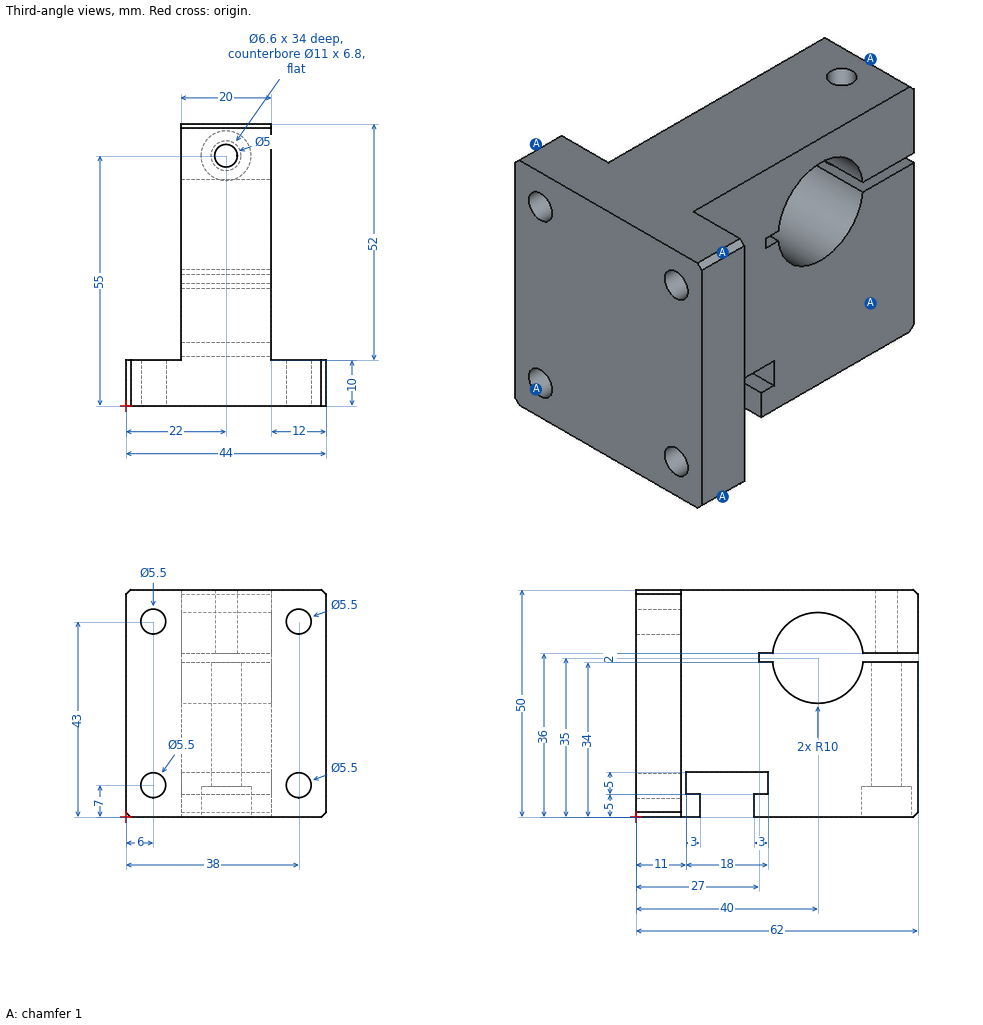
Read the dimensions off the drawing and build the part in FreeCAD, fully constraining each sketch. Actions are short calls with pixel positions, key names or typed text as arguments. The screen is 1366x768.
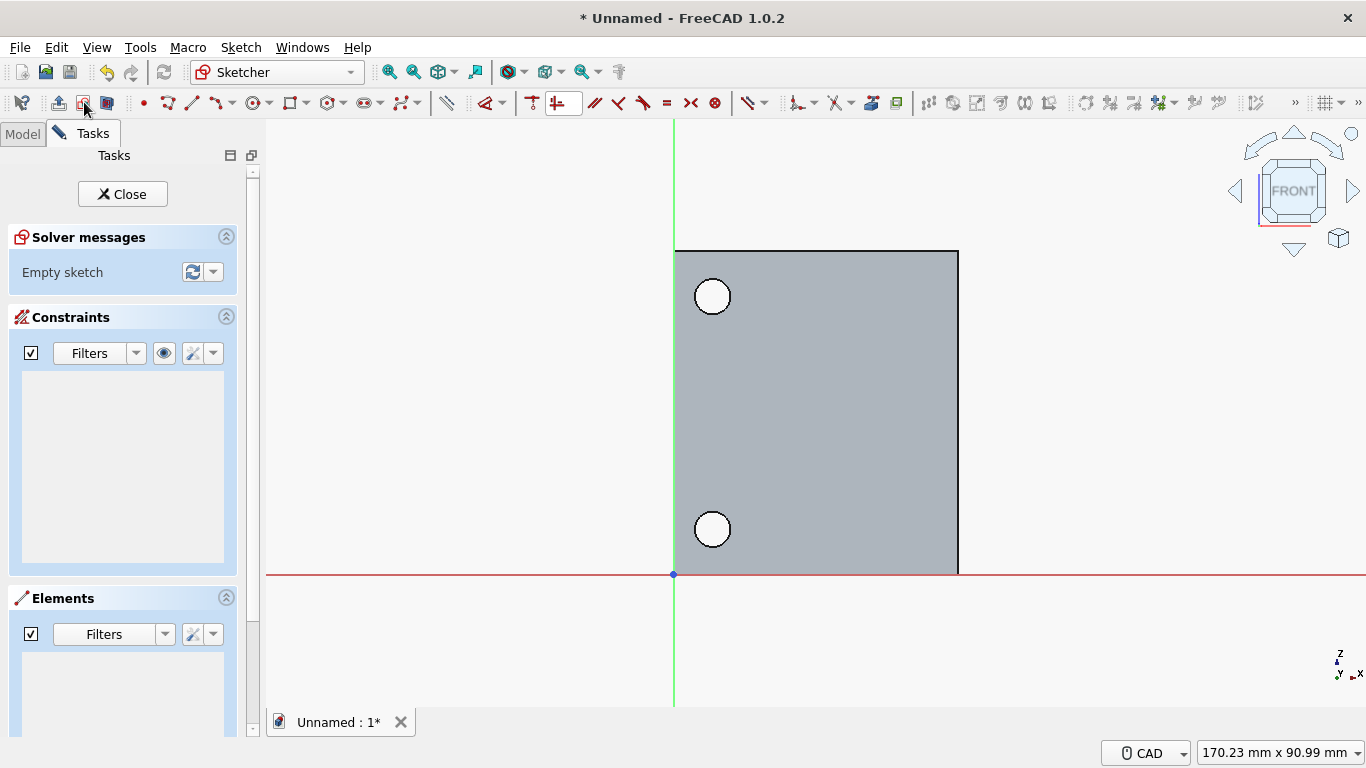
scroll(937, 285, up, 12)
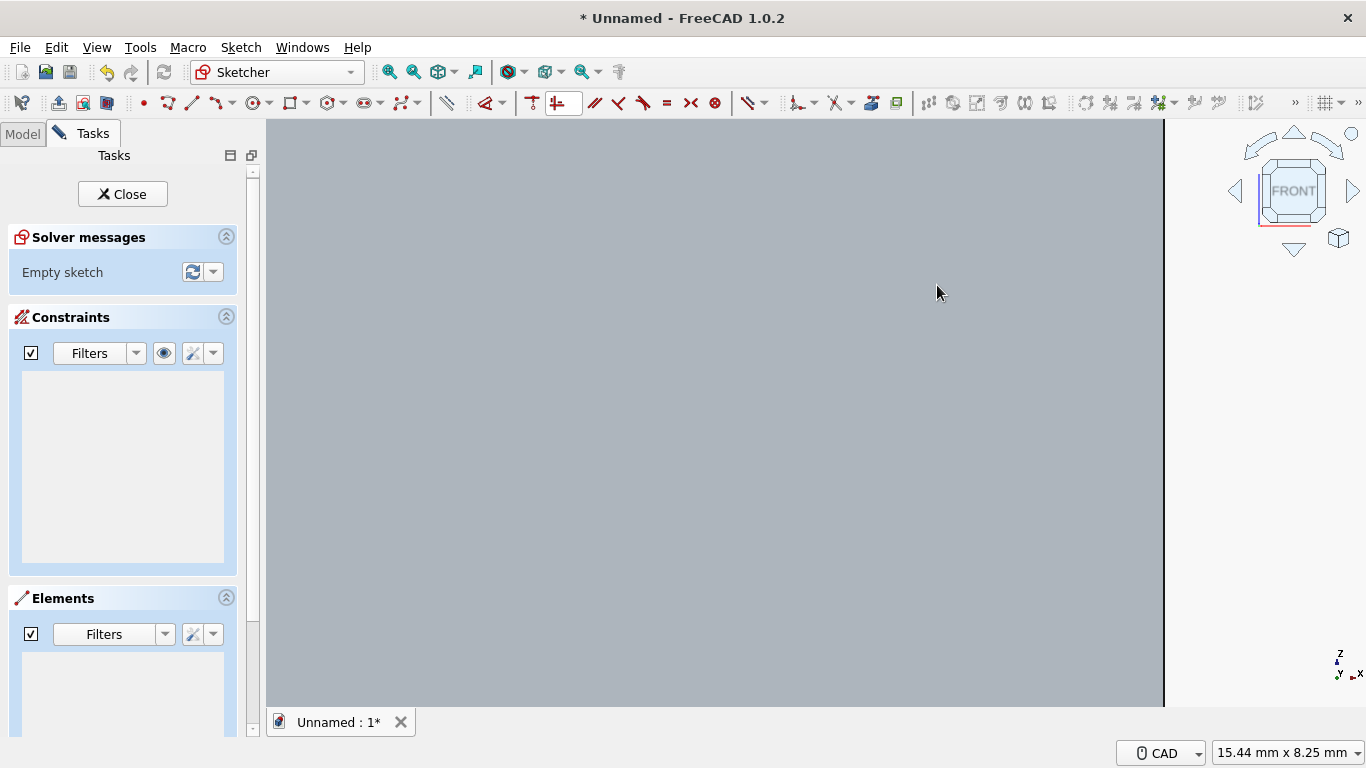
click(254, 104)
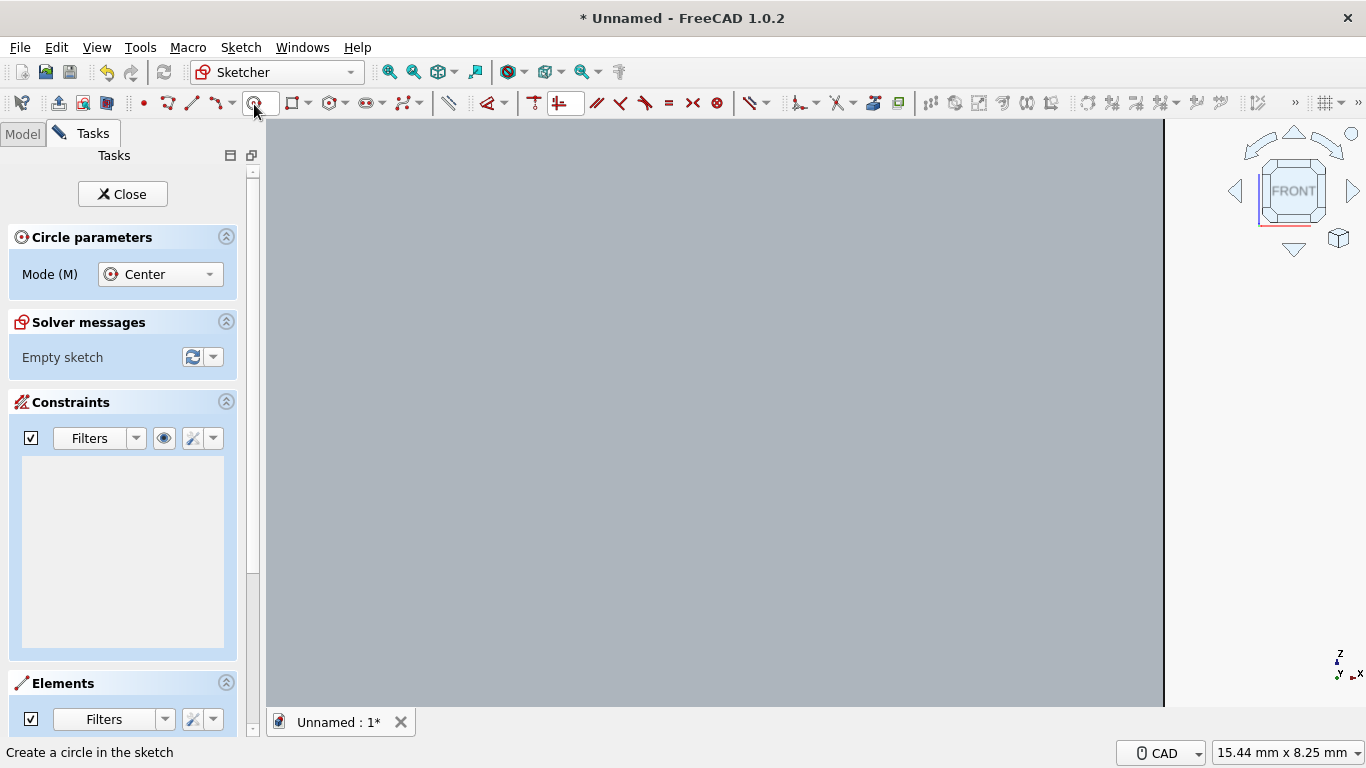
click(737, 411)
move(875, 272)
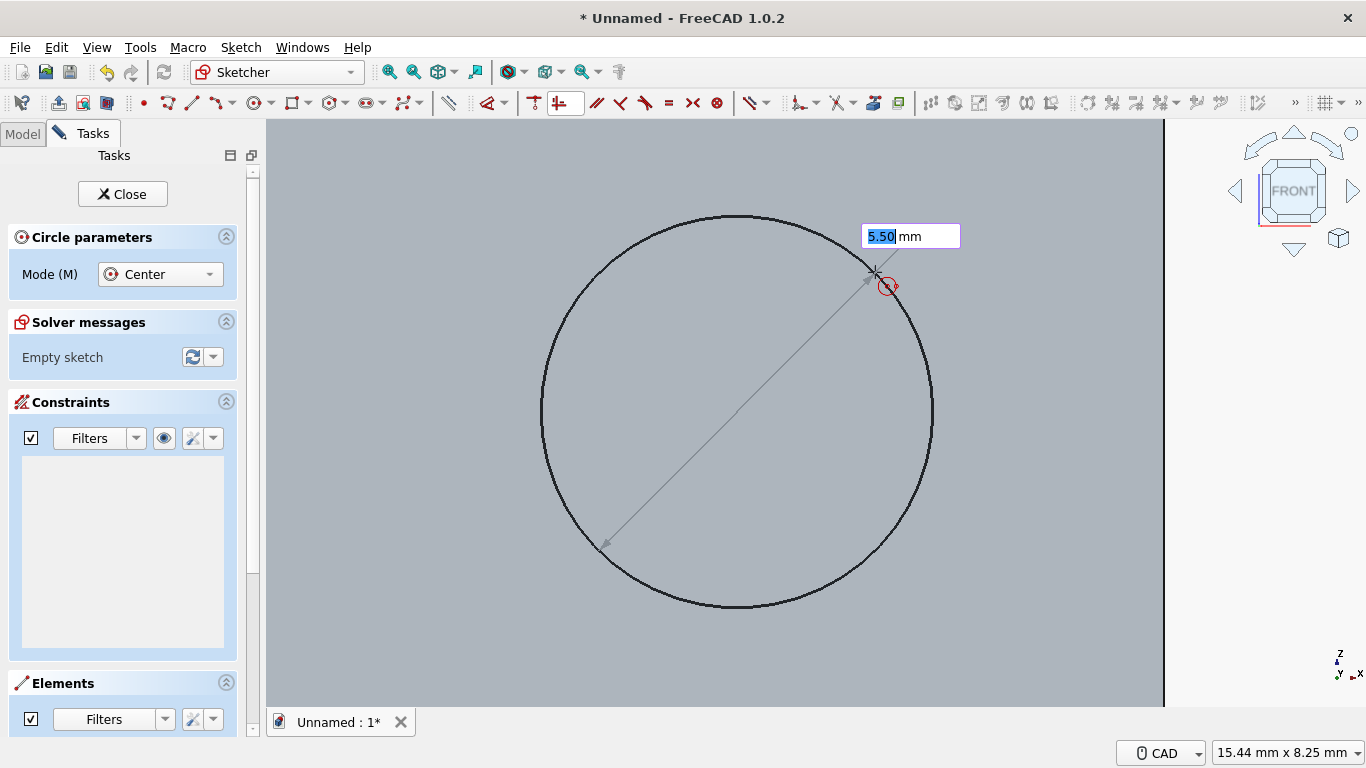
text(5.5)
key(Return)
key(Escape)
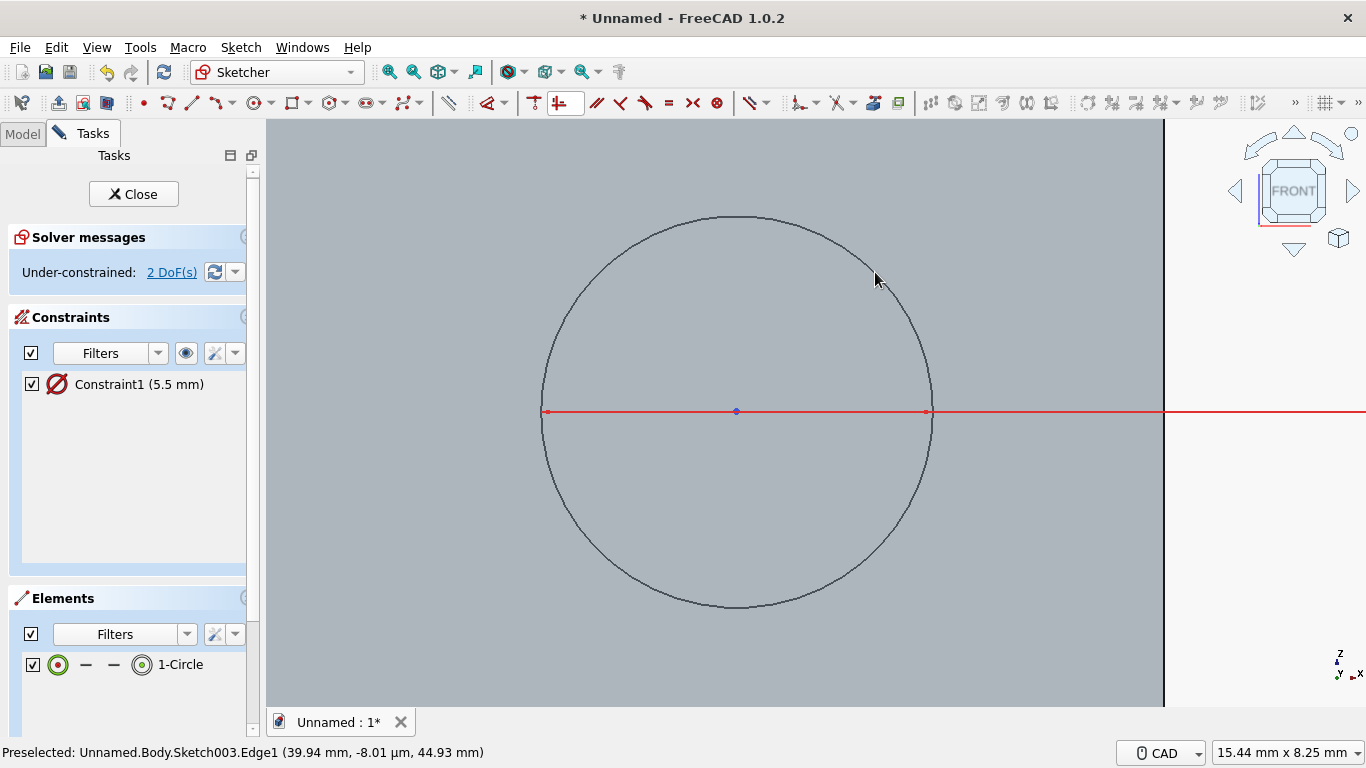
click(488, 104)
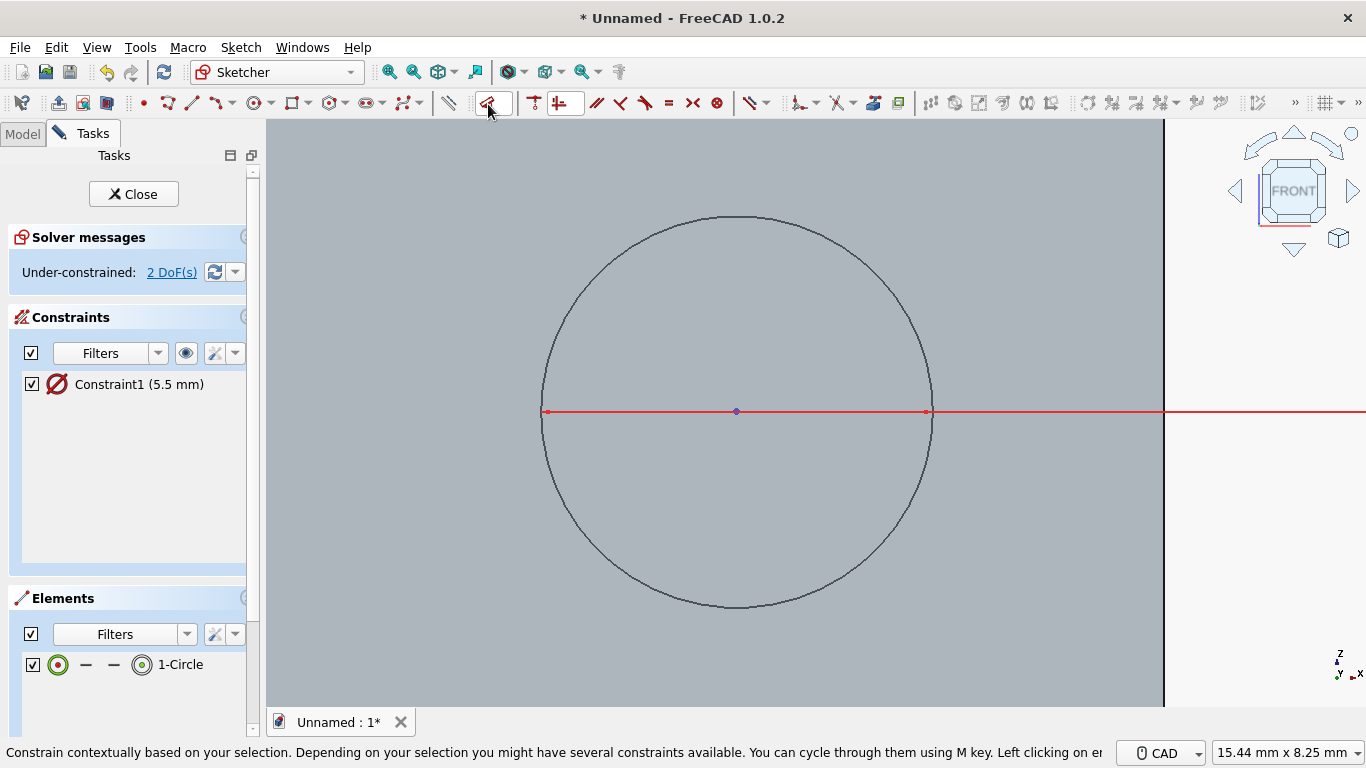
click(737, 412)
click(515, 378)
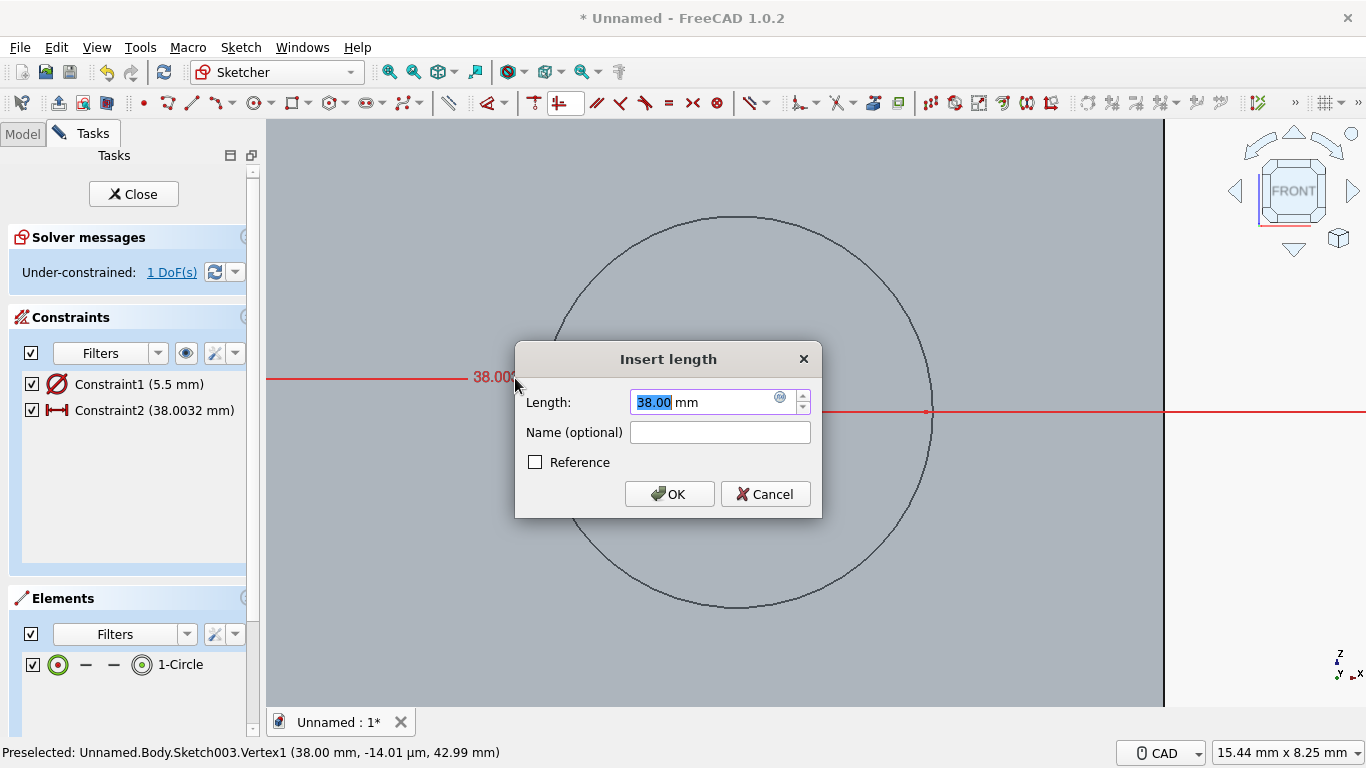
text(38)
key(Return)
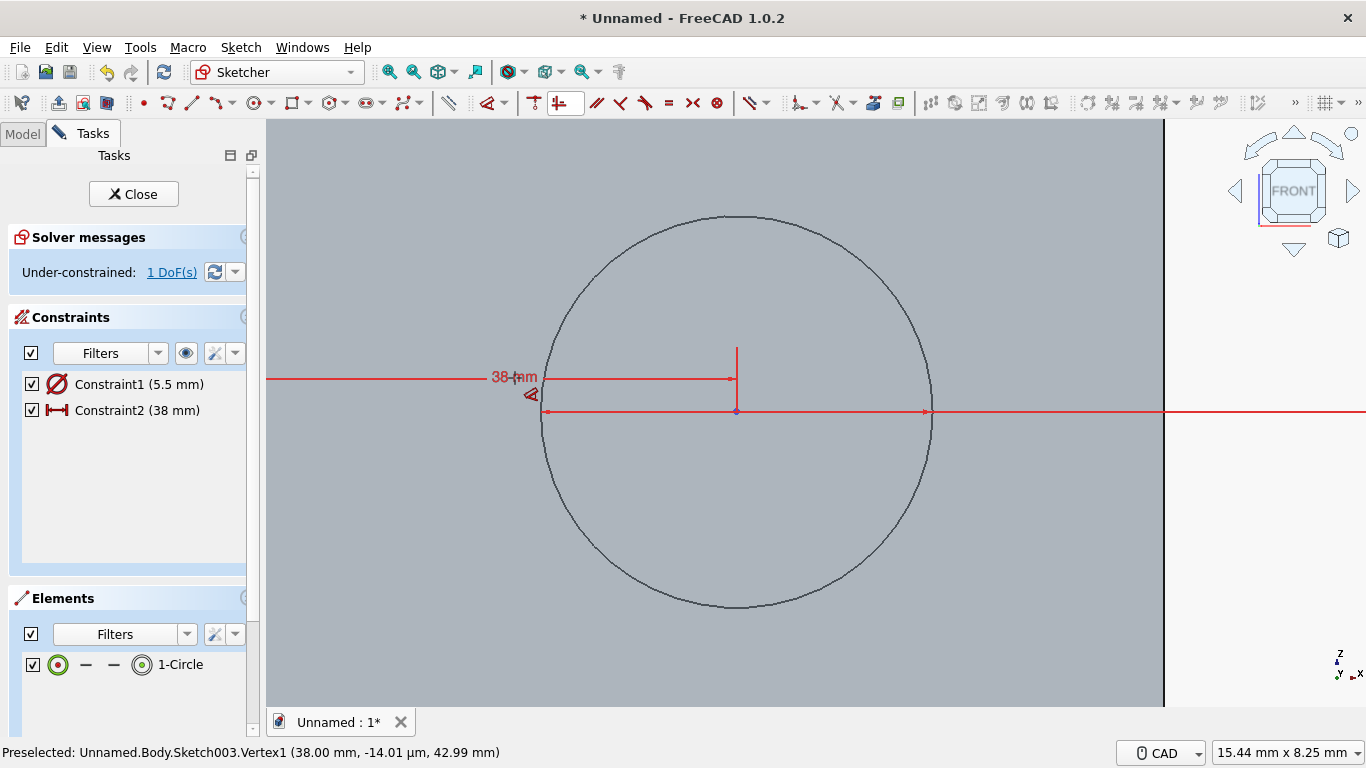
click(737, 412)
click(771, 546)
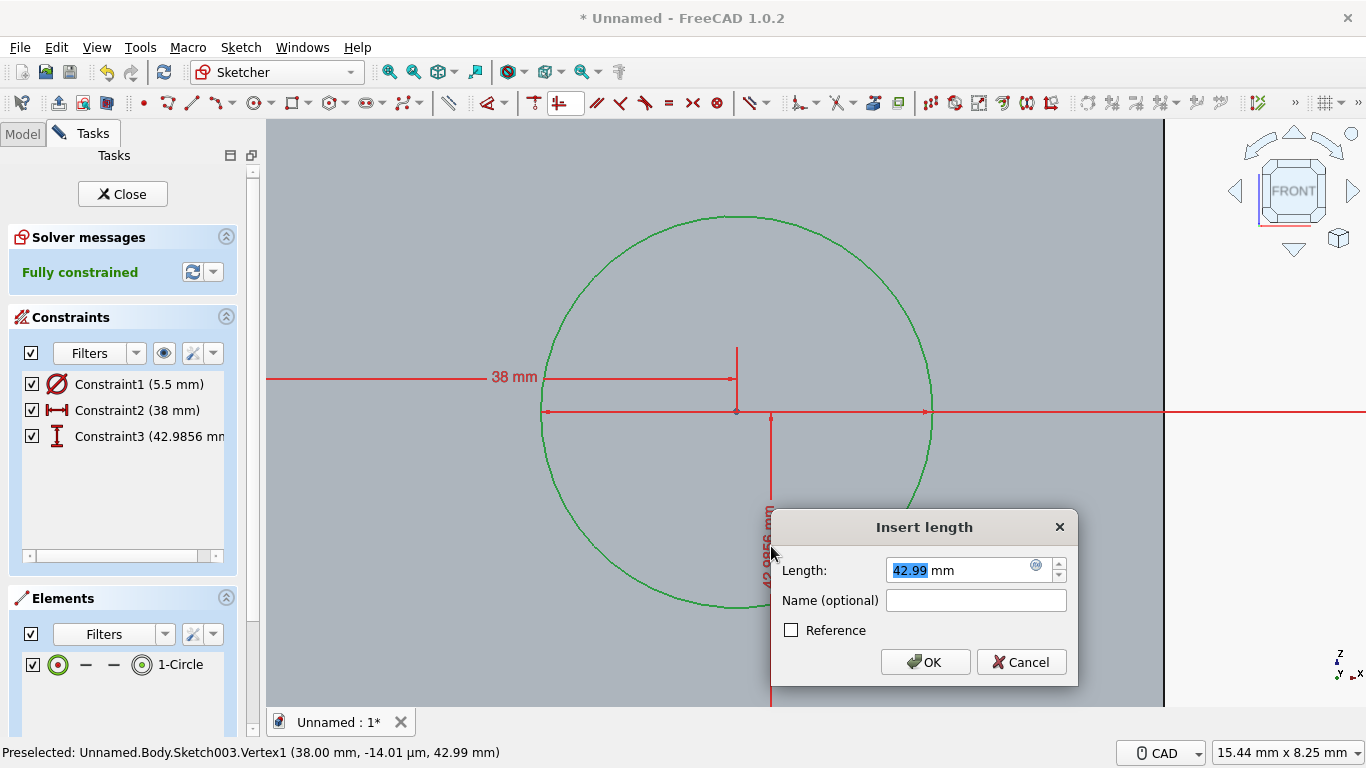
text(43)
key(Return)
key(Escape)